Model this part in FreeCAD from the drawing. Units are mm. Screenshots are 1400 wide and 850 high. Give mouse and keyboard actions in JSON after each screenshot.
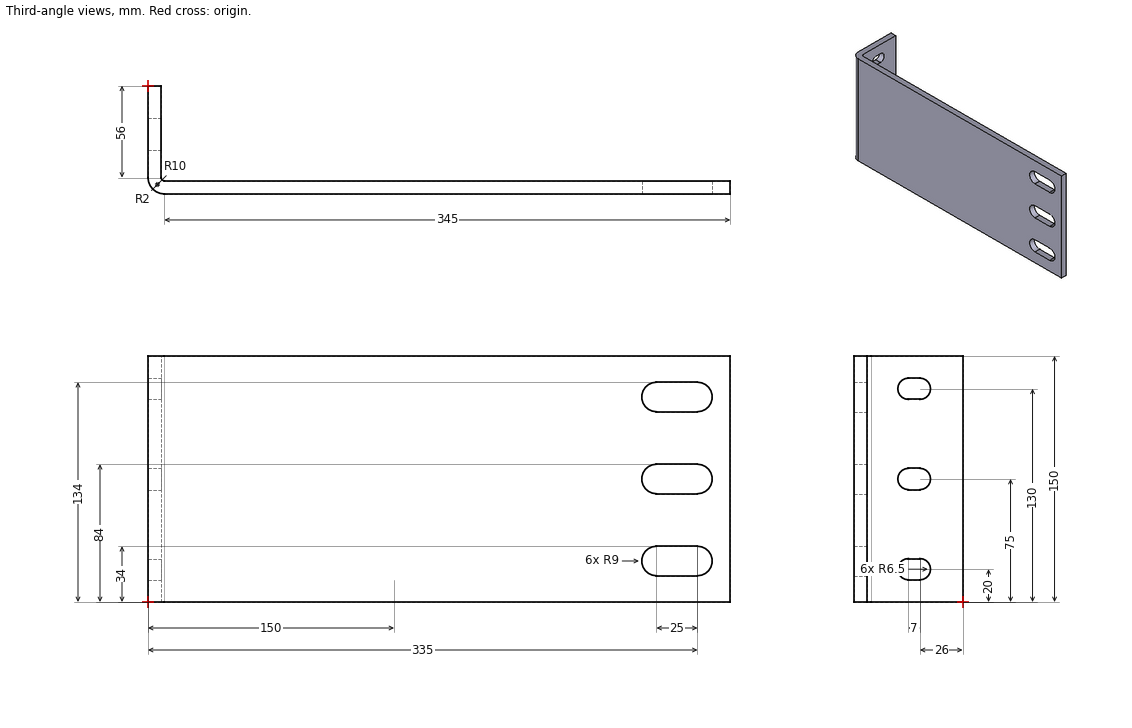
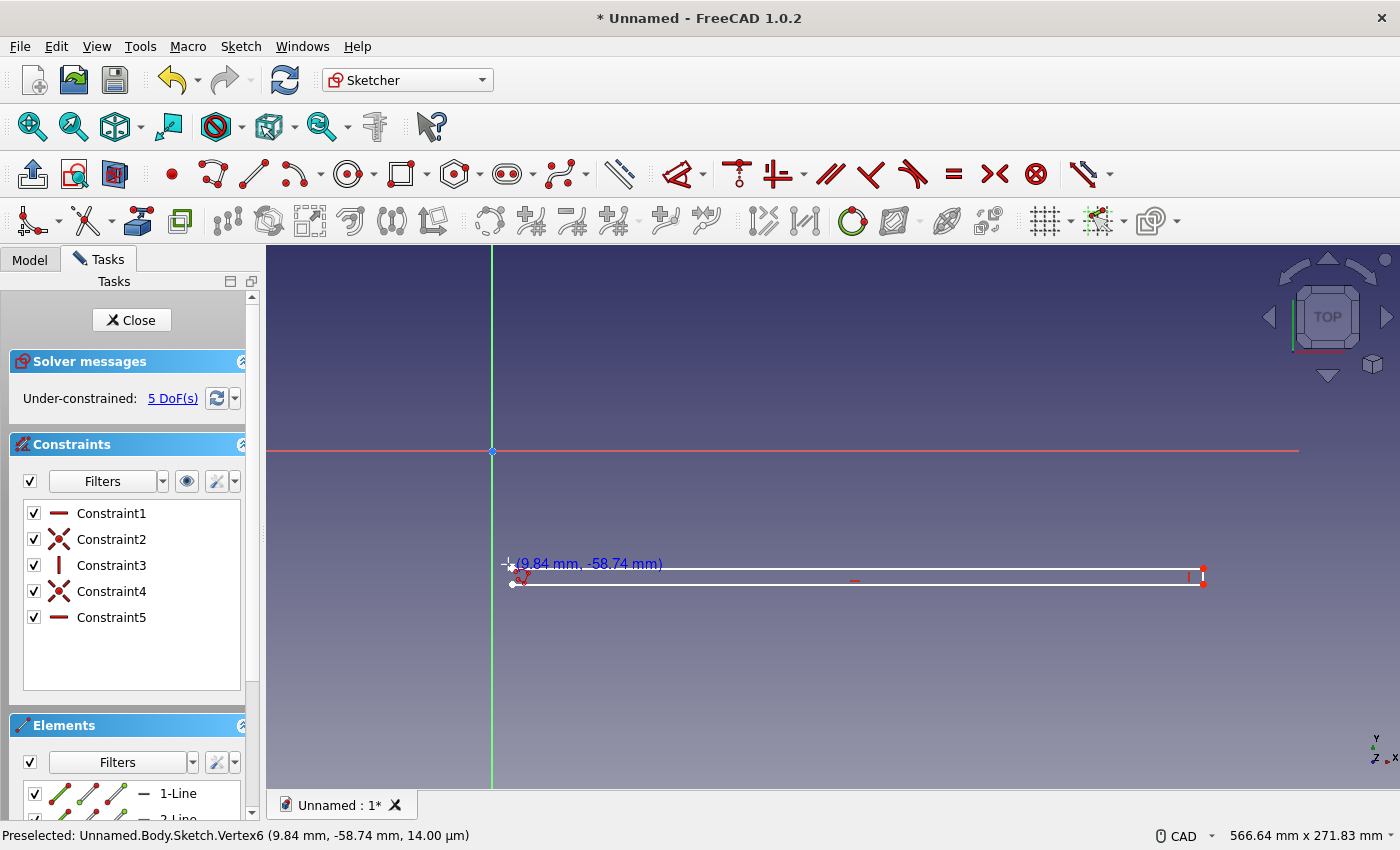
{"action": "left_click", "coordinate": [509, 561]}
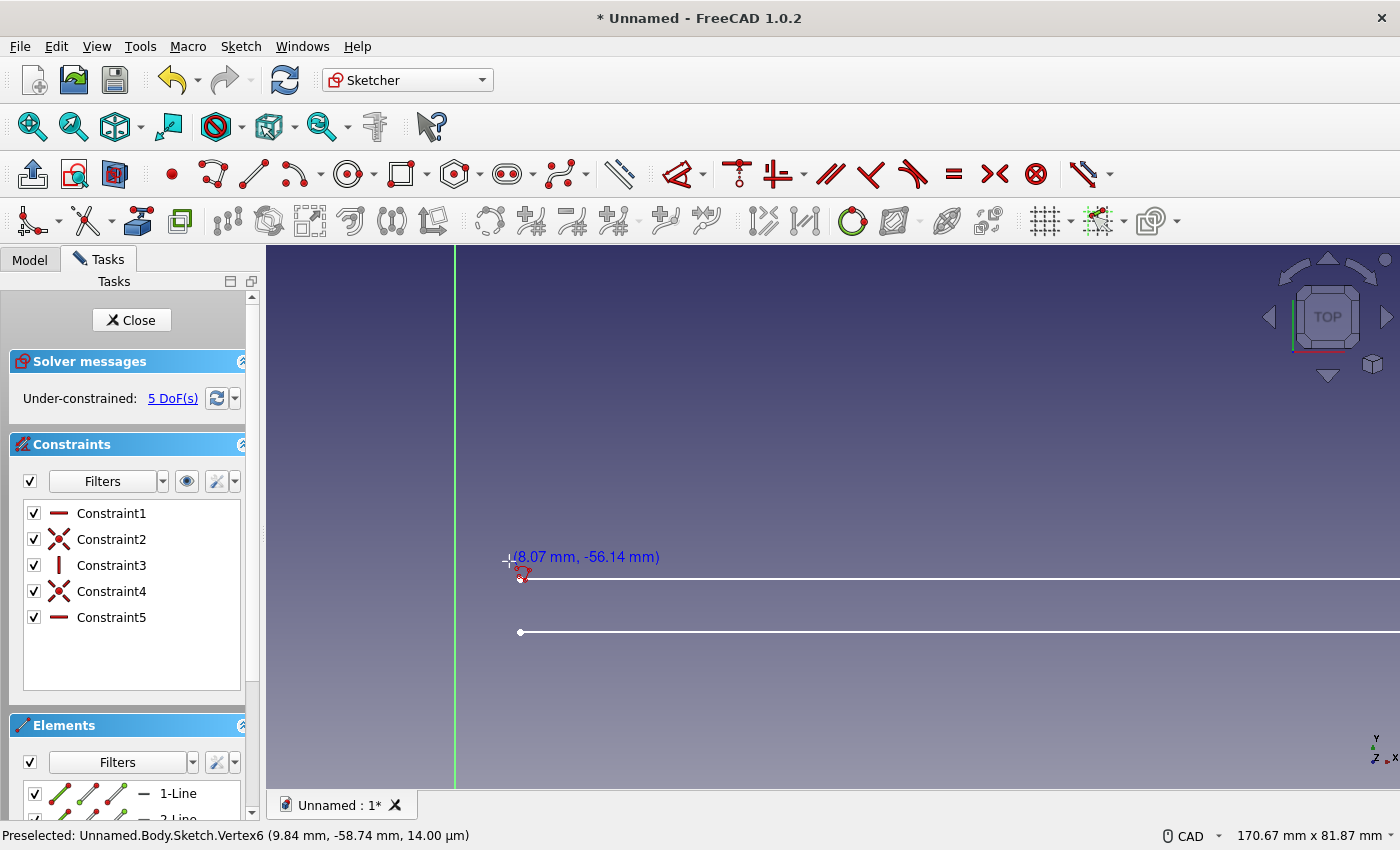
{"action": "scroll", "coordinate": [389, 564], "scroll_direction": "down", "scroll_amount": 6}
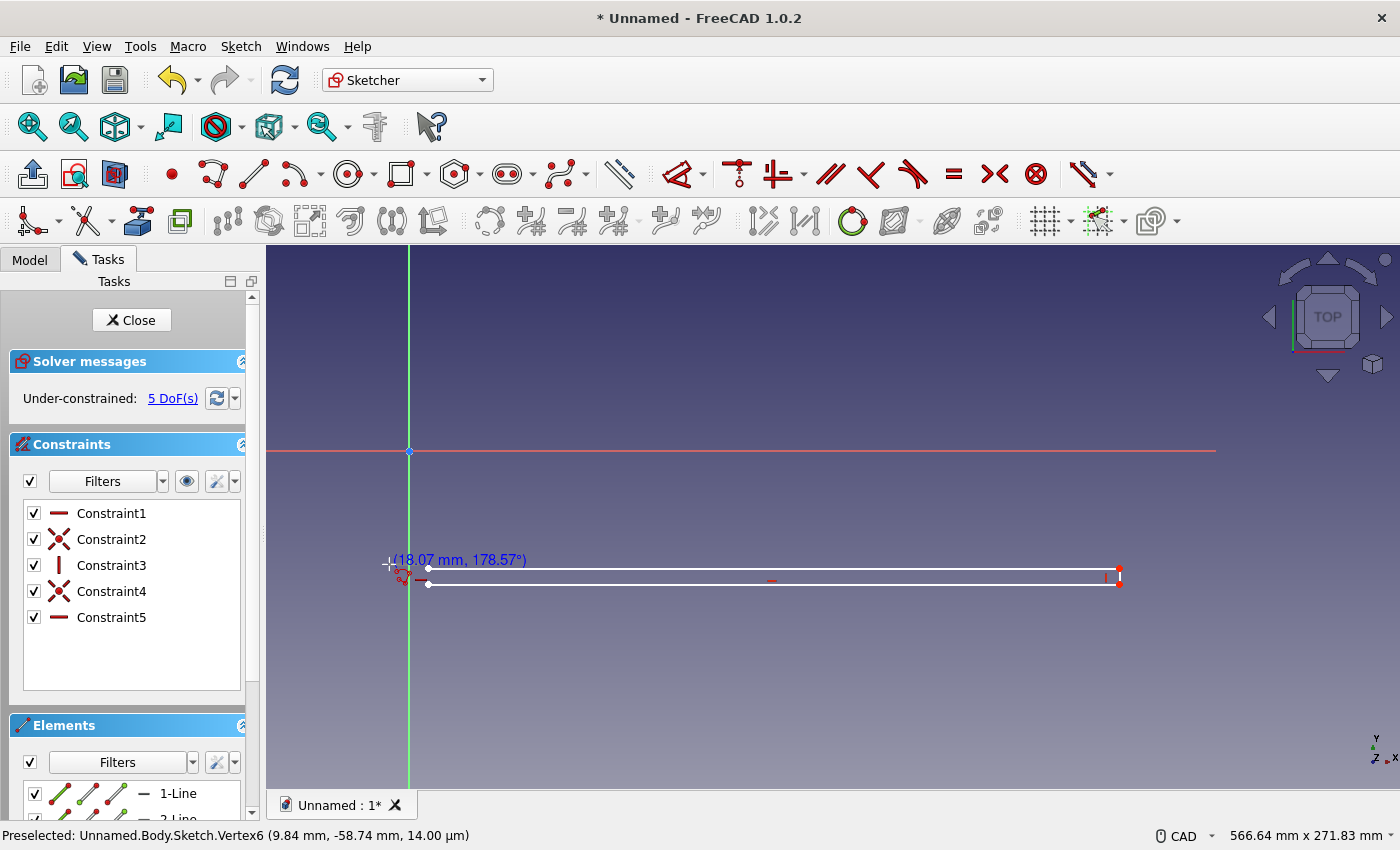
{"action": "left_click", "coordinate": [425, 451]}
{"action": "left_click", "coordinate": [409, 451]}
{"action": "left_click", "coordinate": [418, 564]}
{"action": "right_click", "coordinate": [418, 564]}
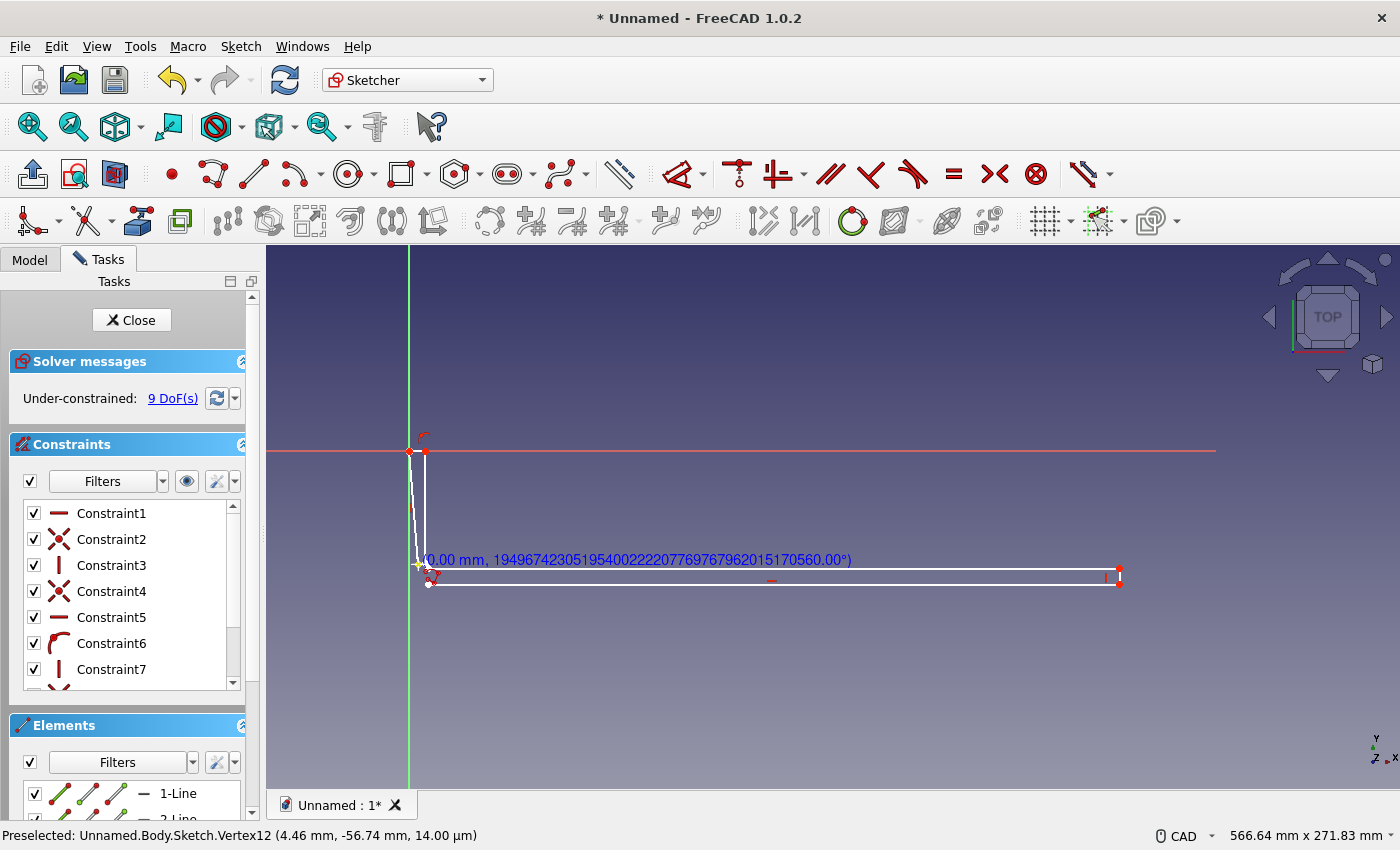
{"action": "left_click", "coordinate": [320, 174]}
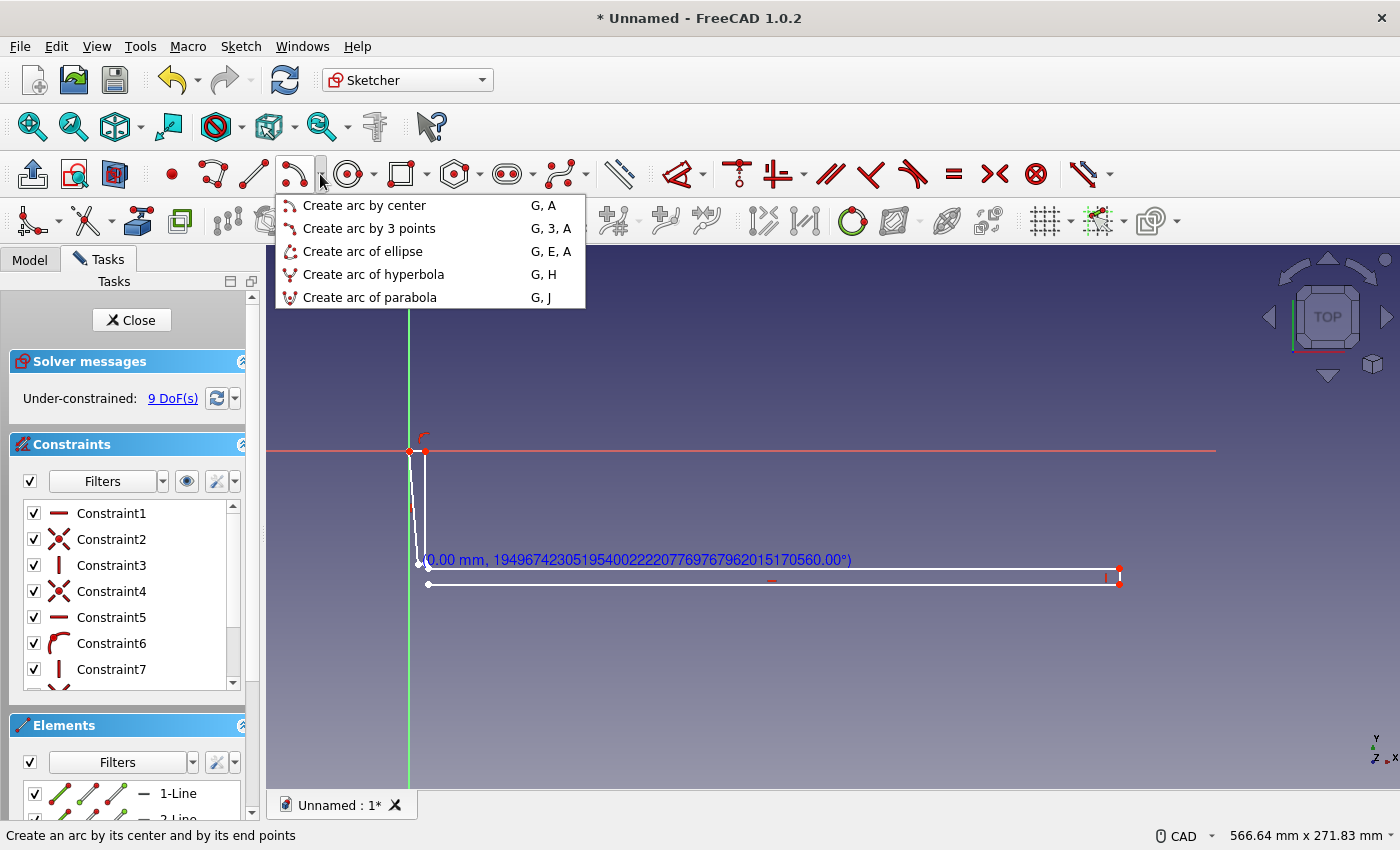
{"action": "left_click", "coordinate": [430, 228]}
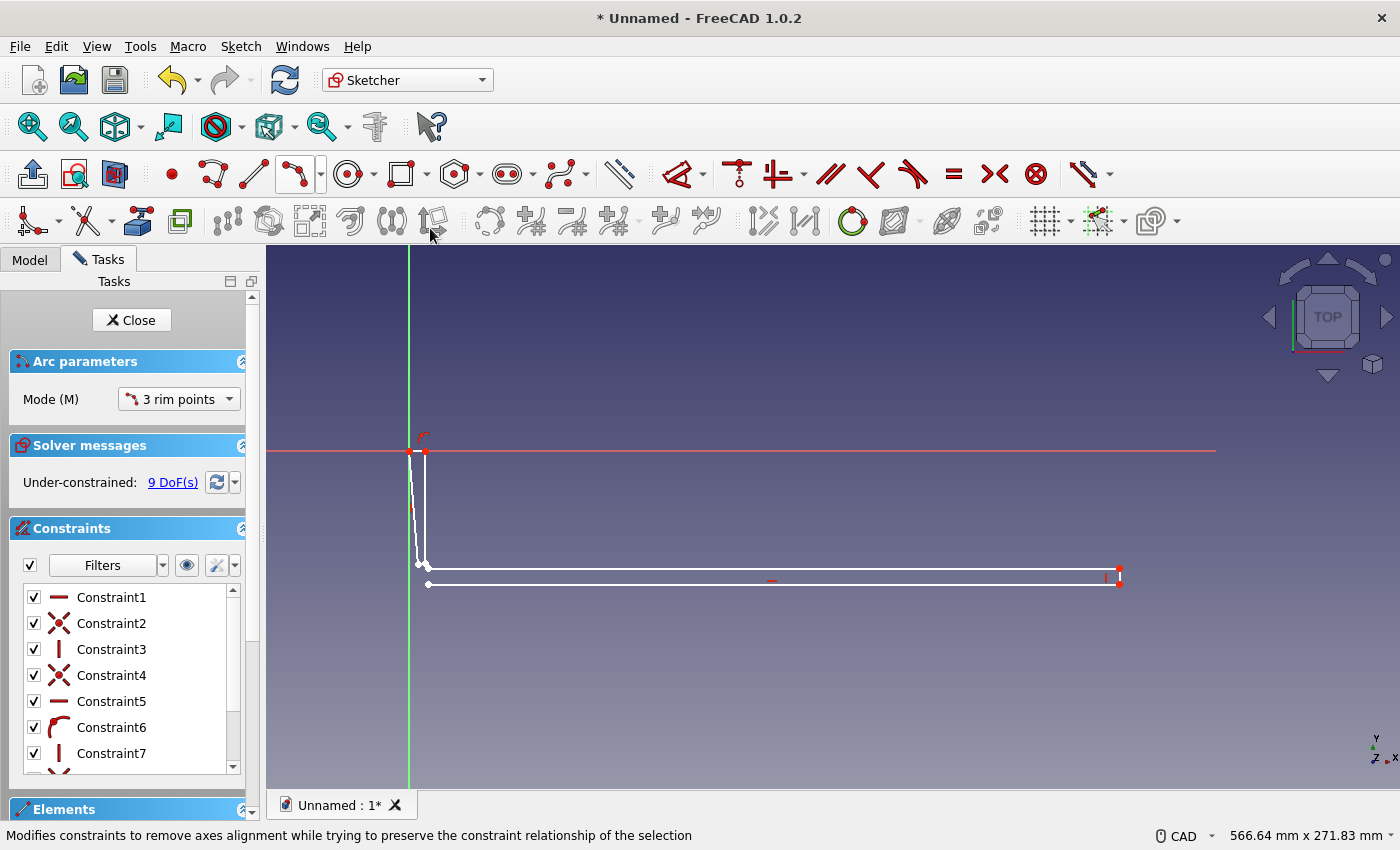
{"action": "scroll", "coordinate": [429, 568], "scroll_direction": "up", "scroll_amount": 6}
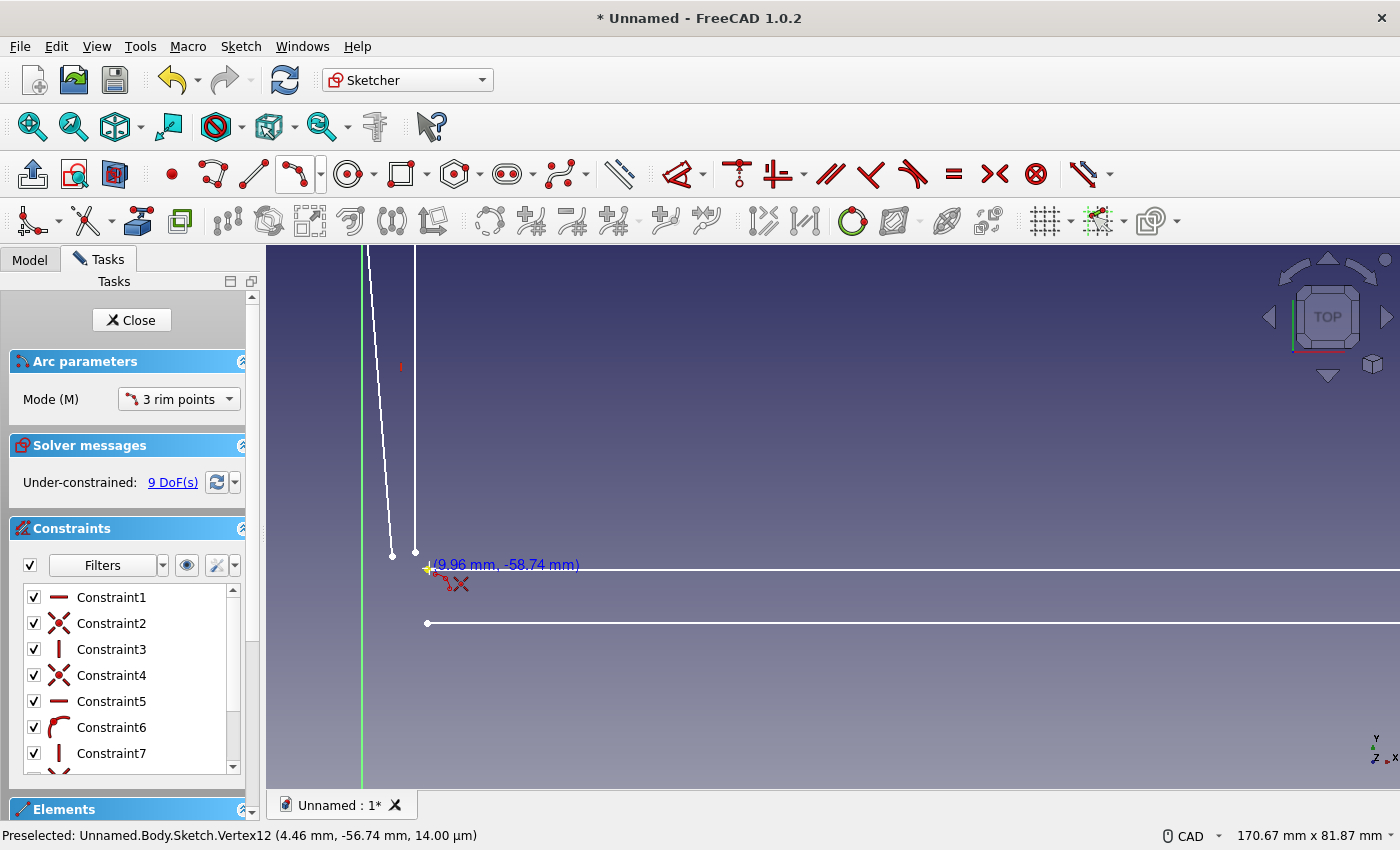
{"action": "left_click", "coordinate": [428, 570]}
{"action": "left_click", "coordinate": [415, 553]}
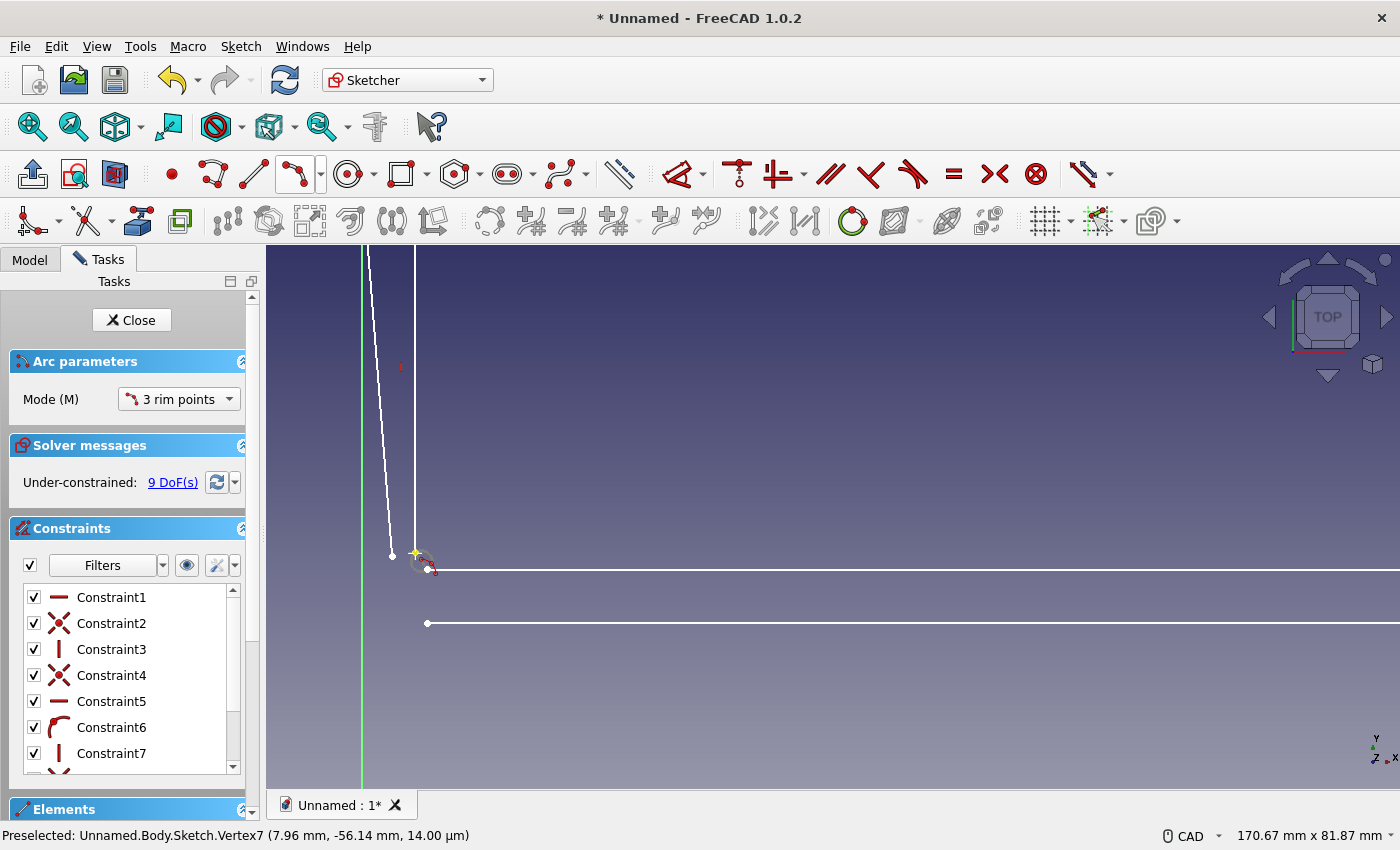
{"action": "scroll", "coordinate": [420, 561], "scroll_direction": "up", "scroll_amount": 8}